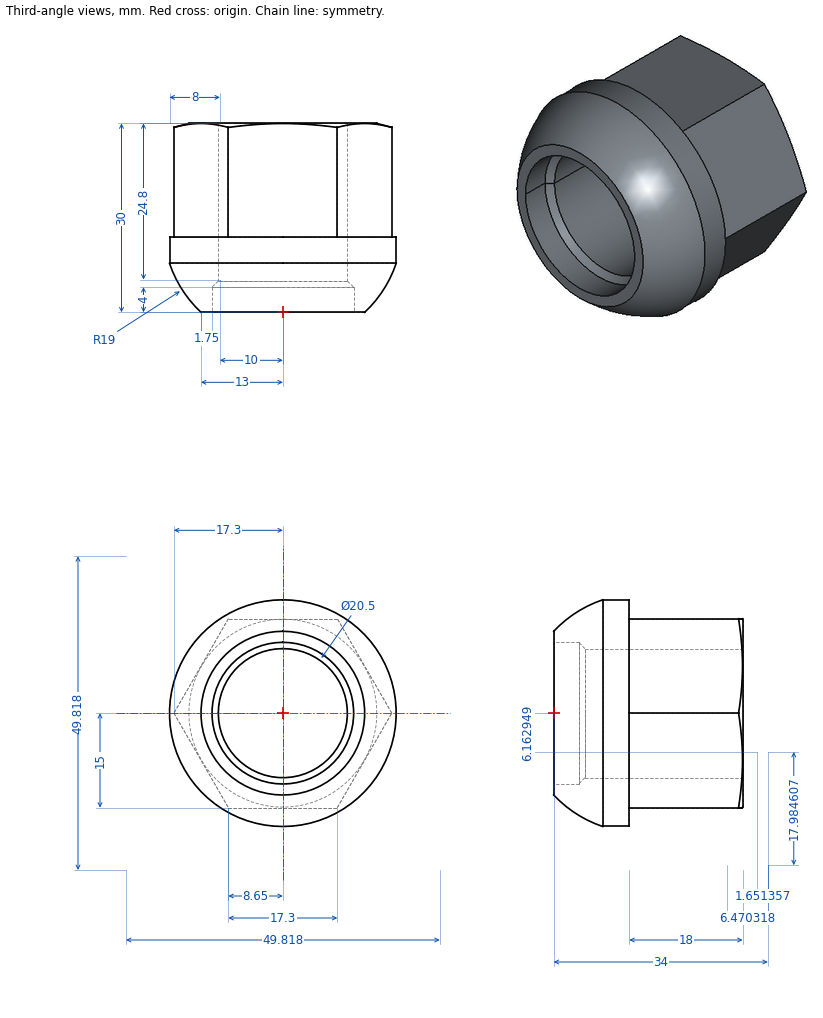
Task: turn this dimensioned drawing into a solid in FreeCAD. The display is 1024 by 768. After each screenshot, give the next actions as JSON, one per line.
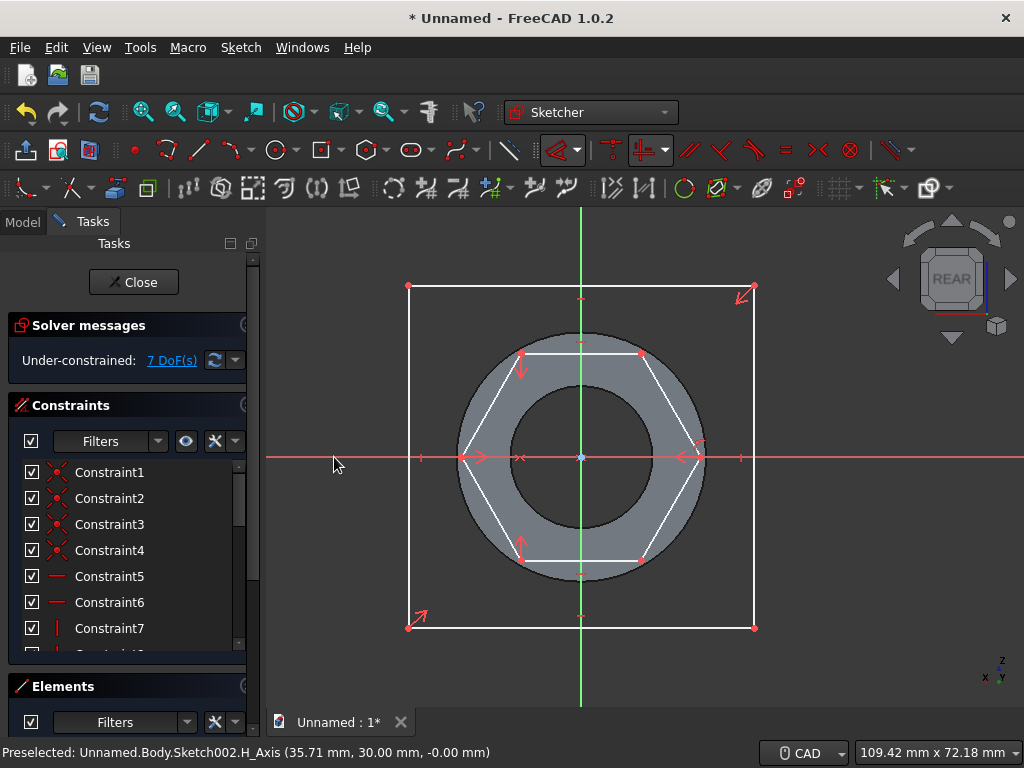
{"action": "left_click", "coordinate": [641, 561]}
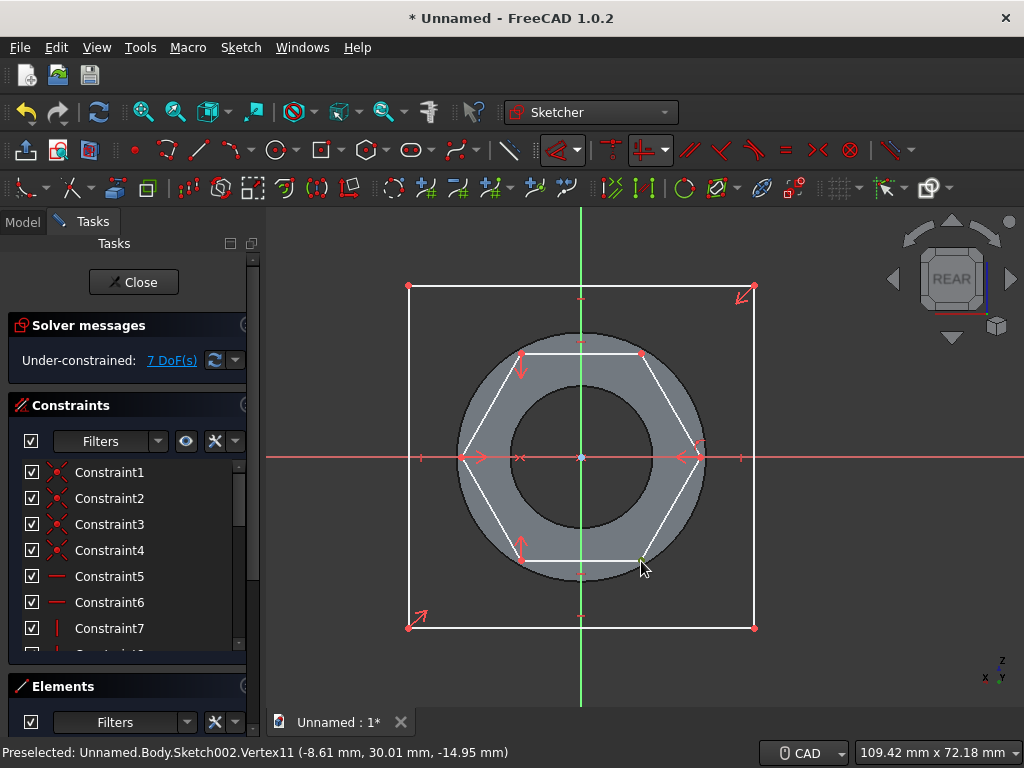
{"action": "key", "text": "i"}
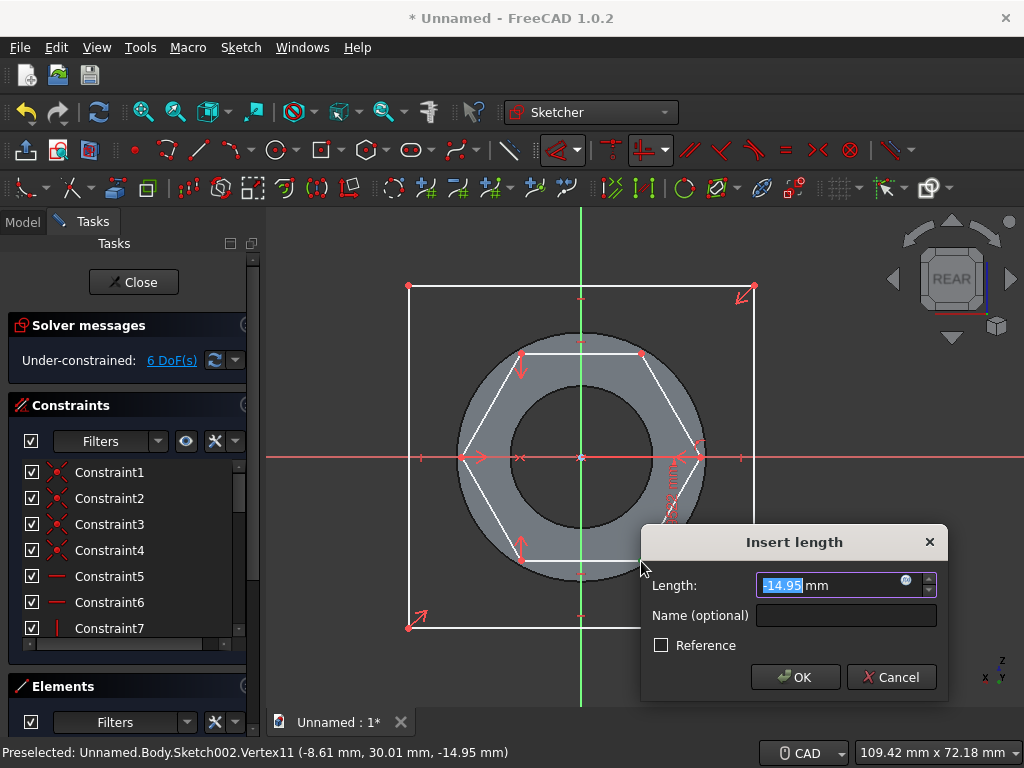
{"action": "type", "text": "-15"}
{"action": "key", "text": "Return"}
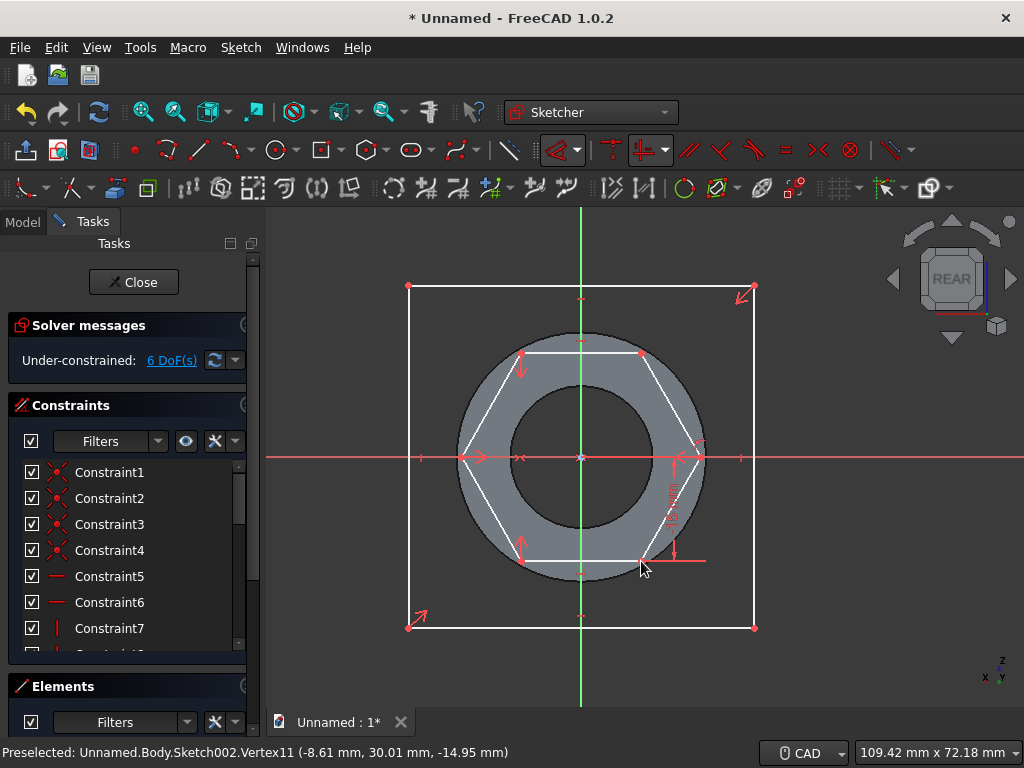
{"action": "left_click", "coordinate": [605, 561]}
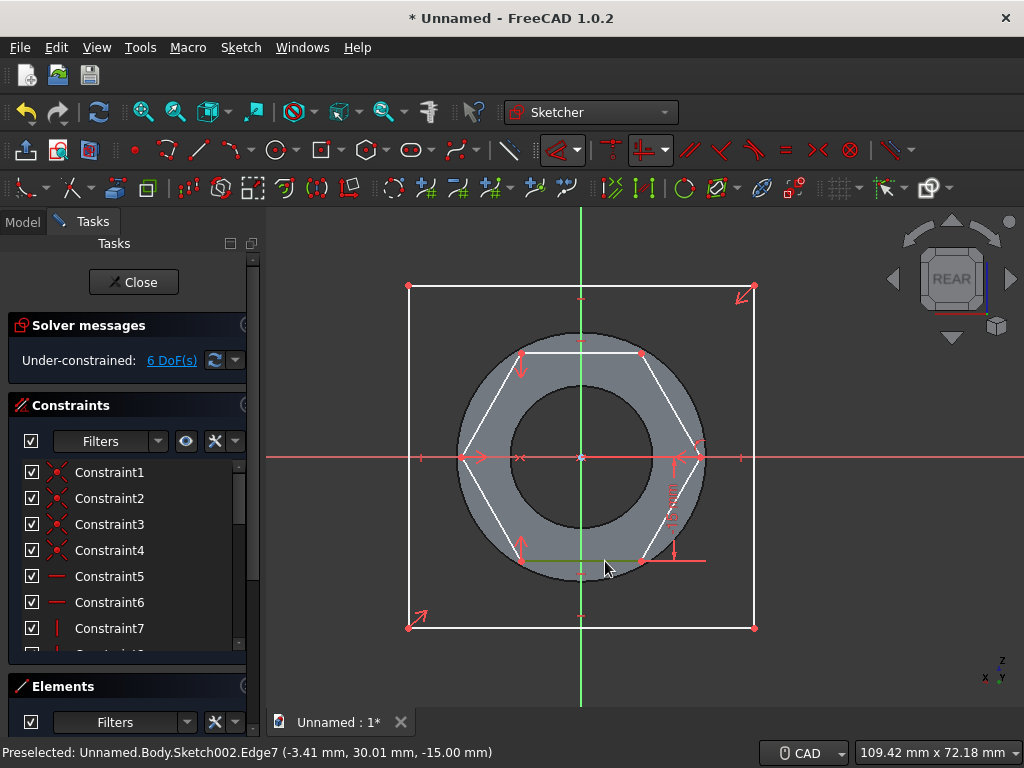
{"action": "key", "text": "l"}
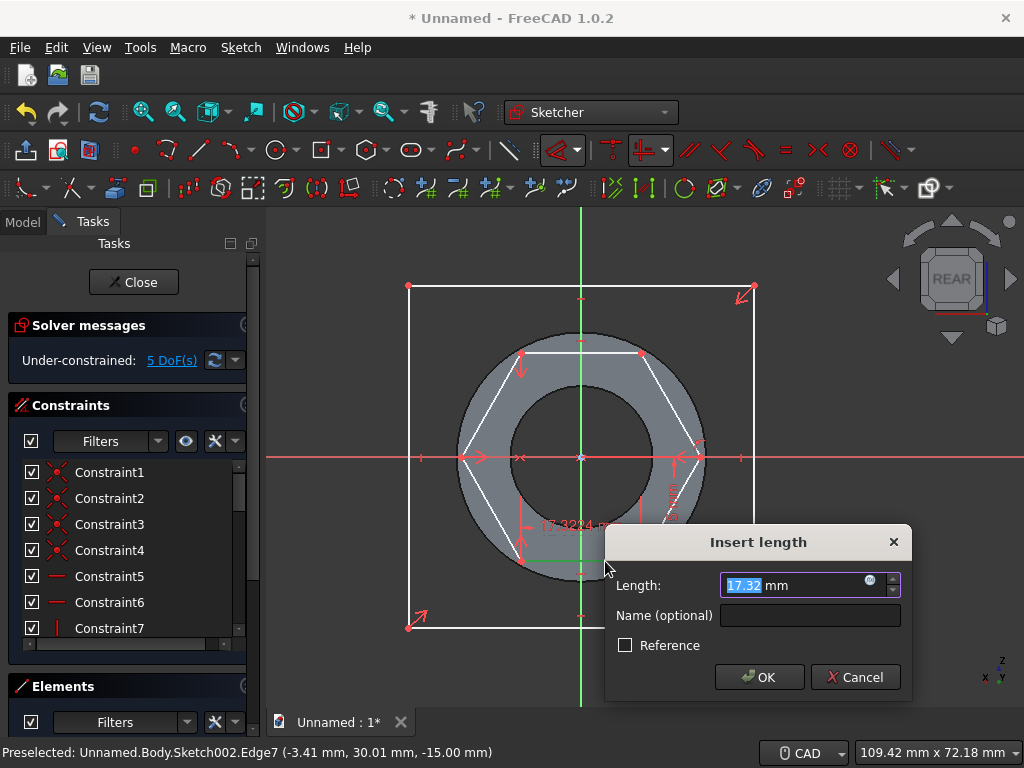
{"action": "type", "text": "17.3"}
{"action": "key", "text": "Return"}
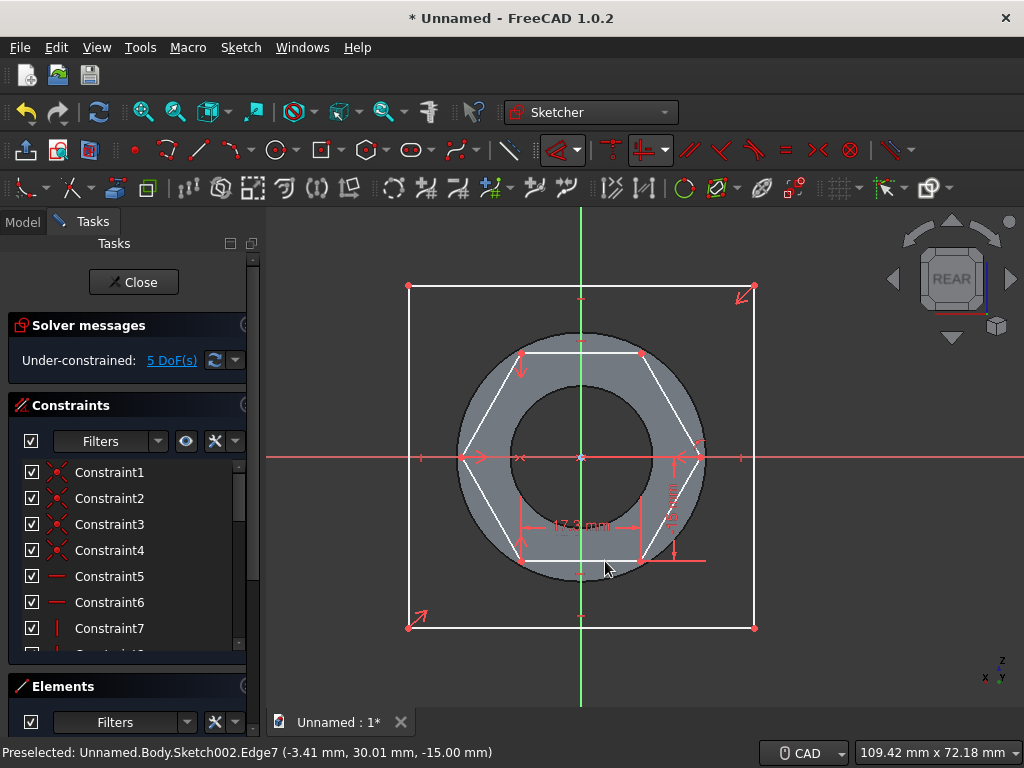
{"action": "left_click", "coordinate": [557, 353]}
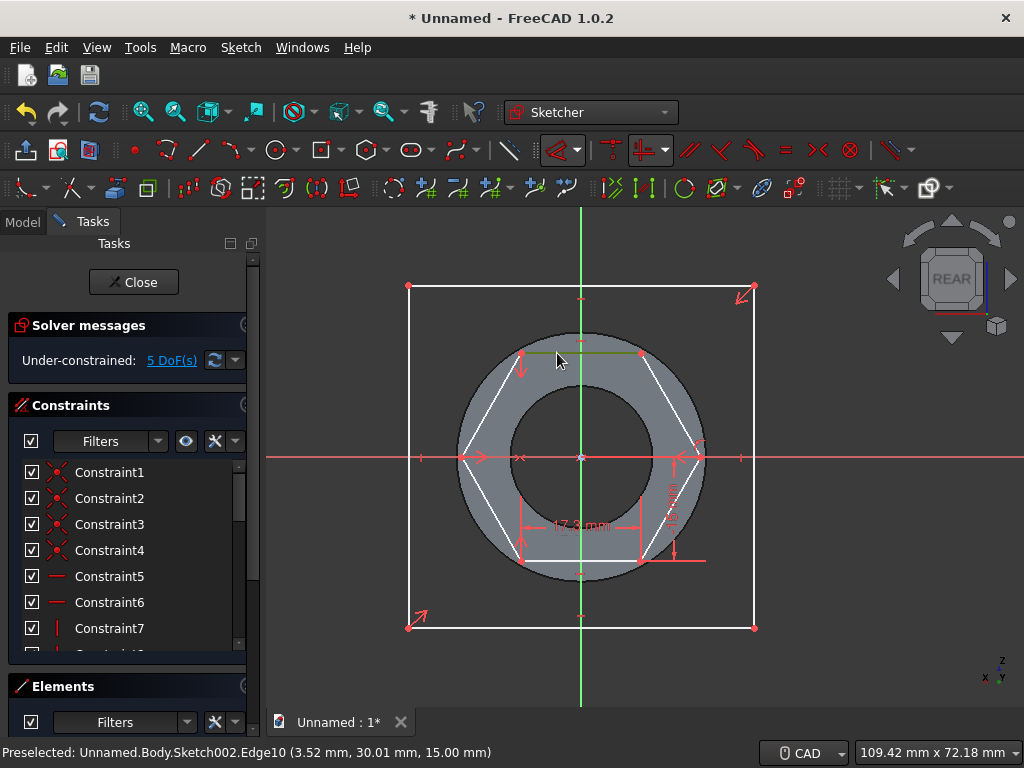
{"action": "key", "text": "l"}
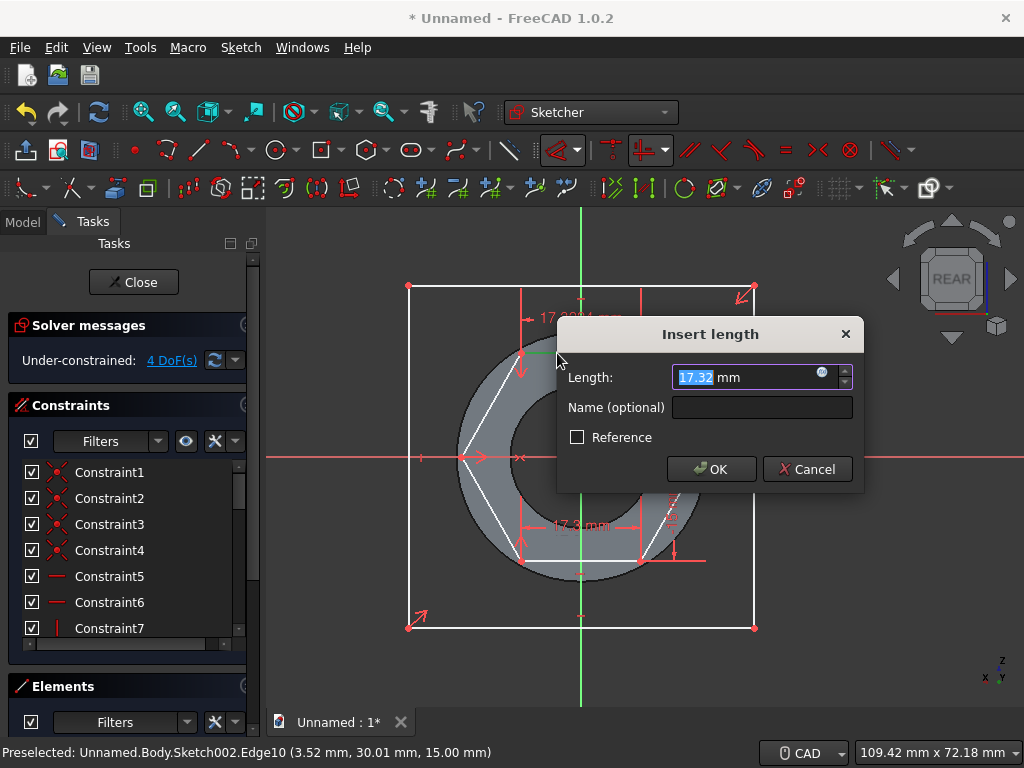
{"action": "type", "text": "17.3"}
{"action": "key", "text": "Return"}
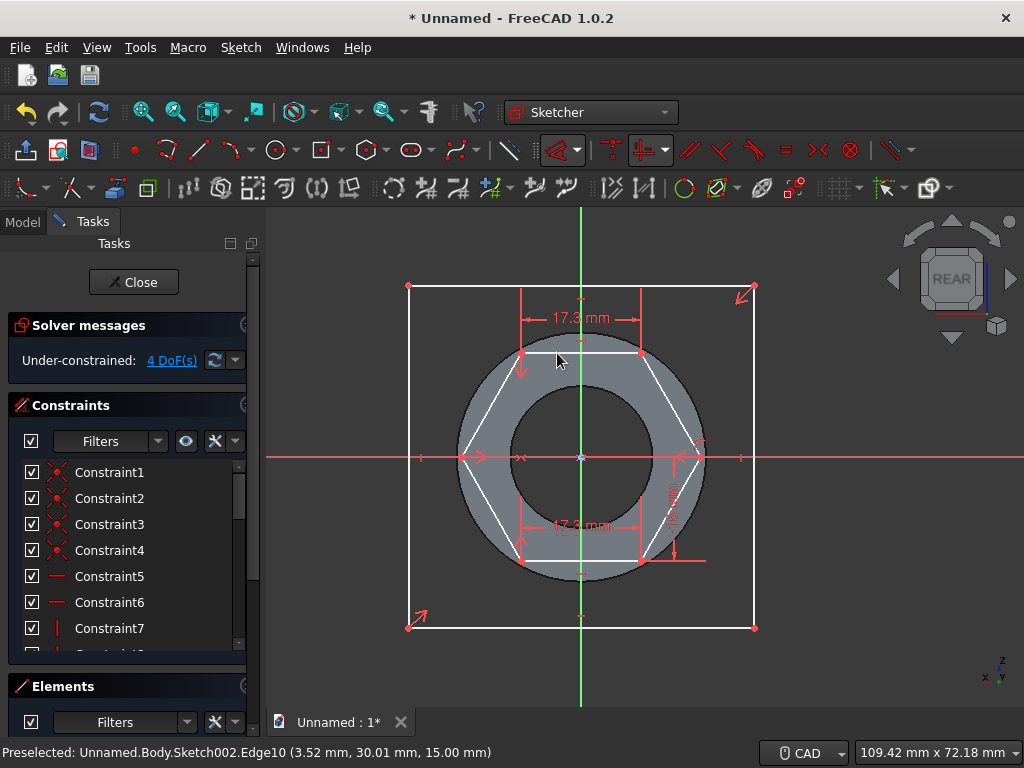
{"action": "left_click", "coordinate": [701, 457]}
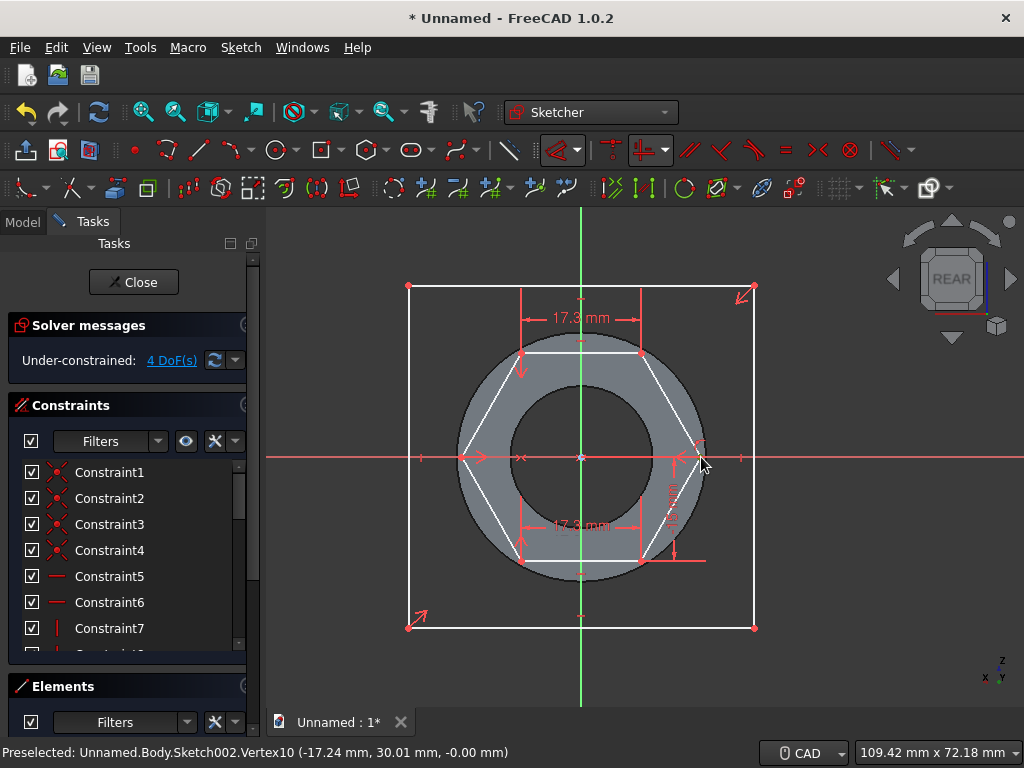
{"action": "left_click", "coordinate": [580, 150]}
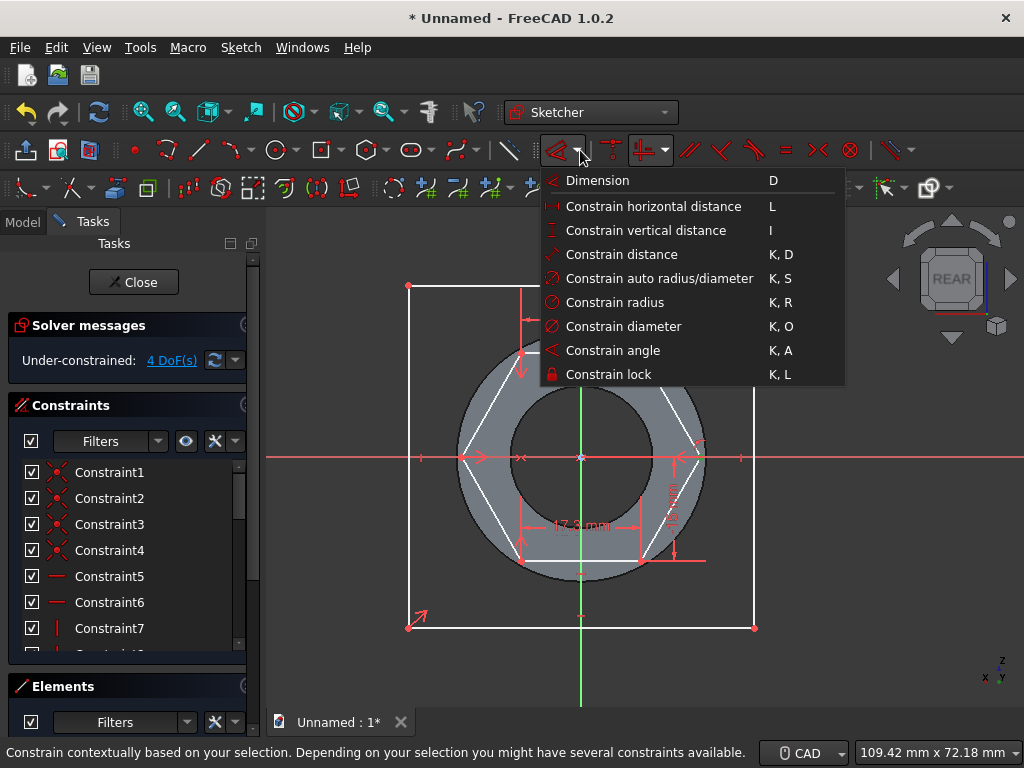
{"action": "left_click", "coordinate": [693, 206]}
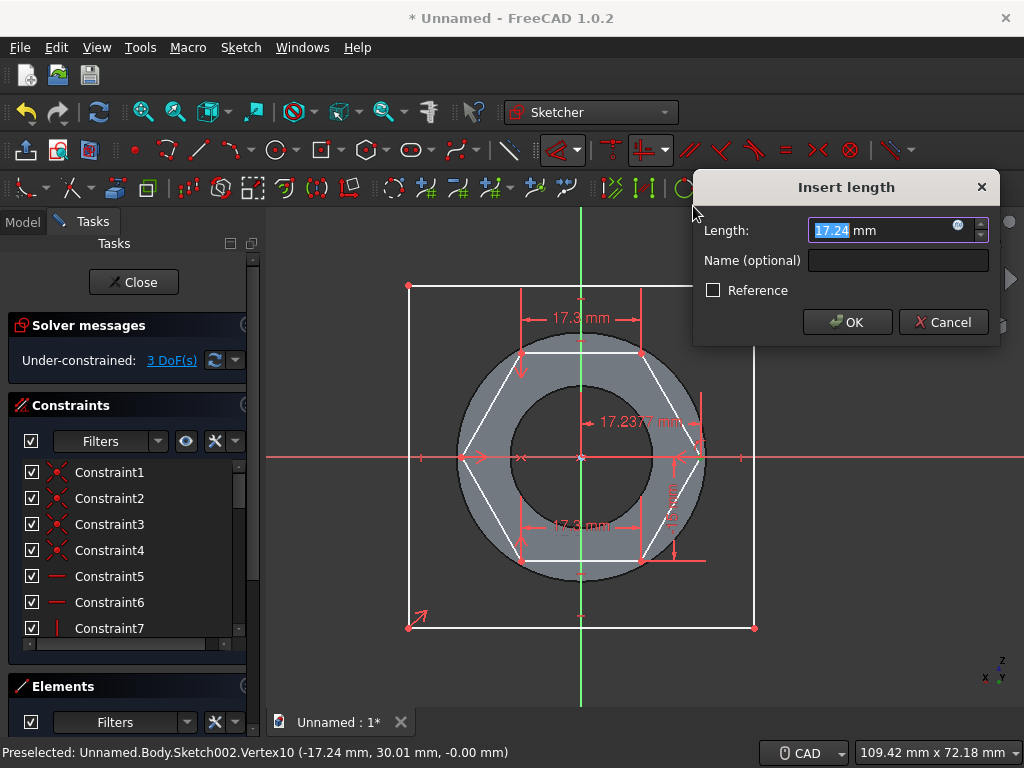
{"action": "type", "text": "17.3"}
{"action": "key", "text": "Return"}